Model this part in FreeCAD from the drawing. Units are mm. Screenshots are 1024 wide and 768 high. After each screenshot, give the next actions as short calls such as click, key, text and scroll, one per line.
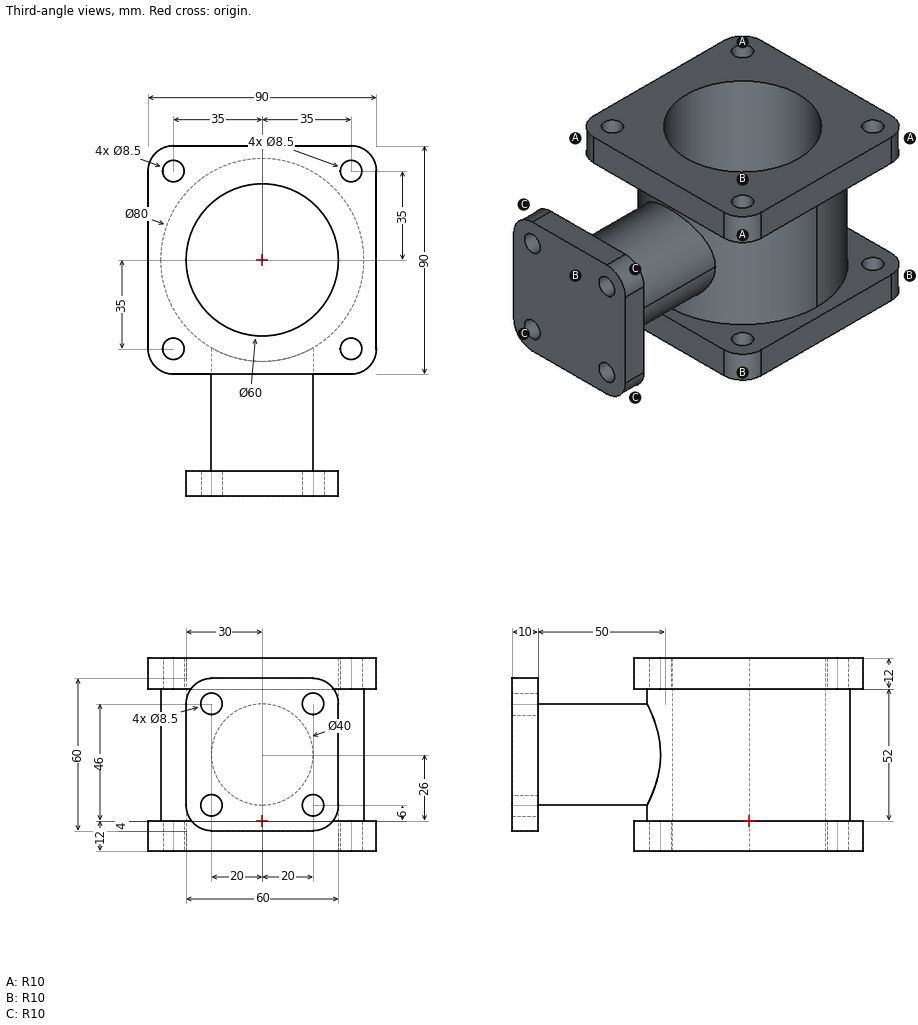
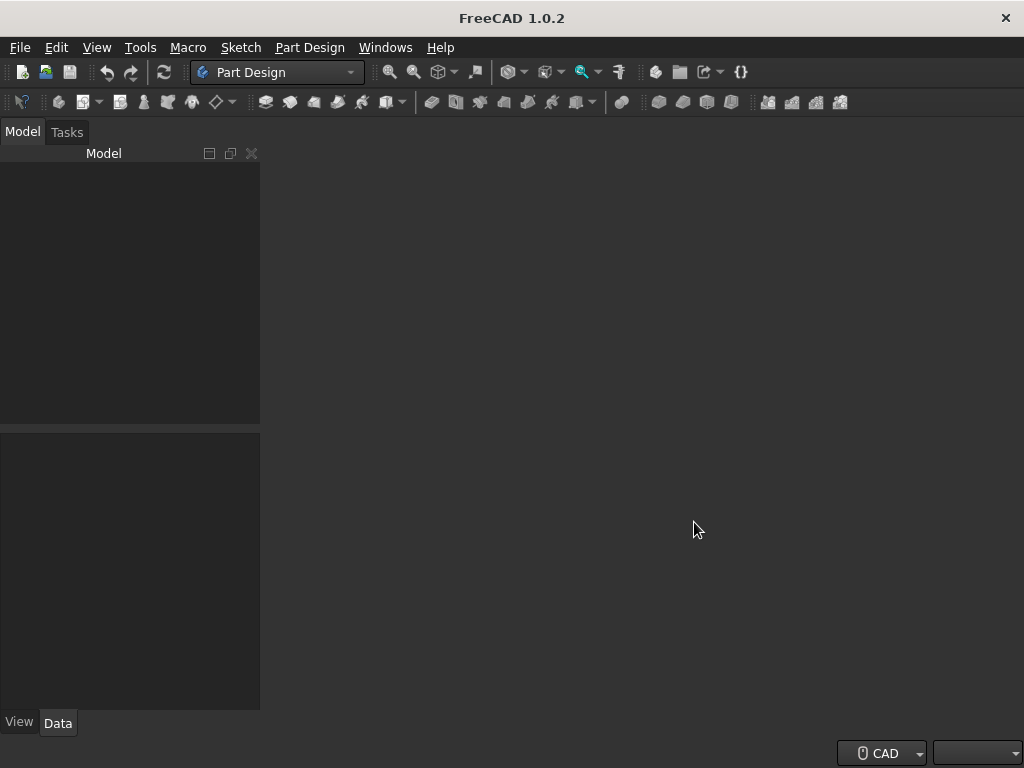
key(ctrl+n)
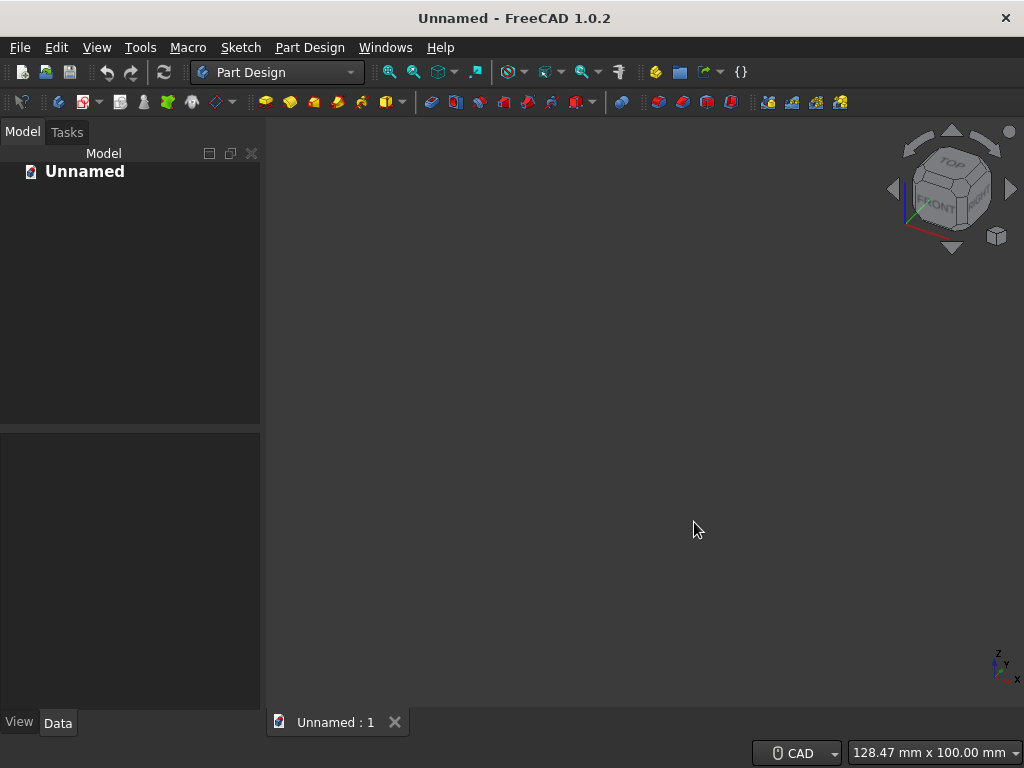
click(84, 102)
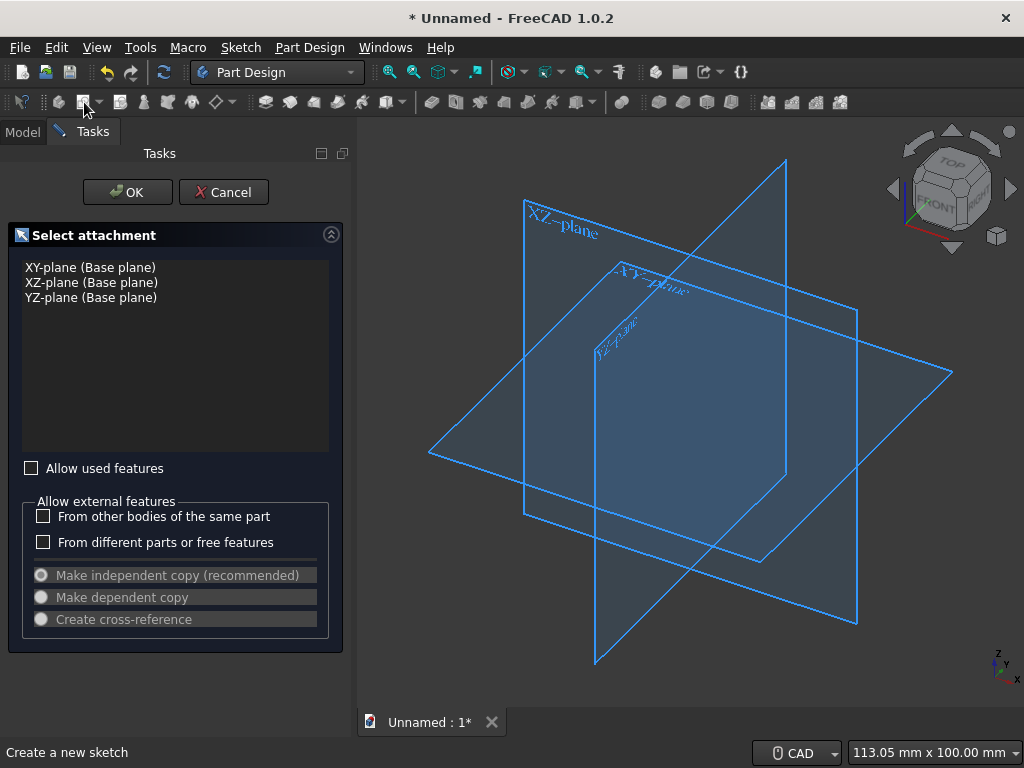
click(82, 268)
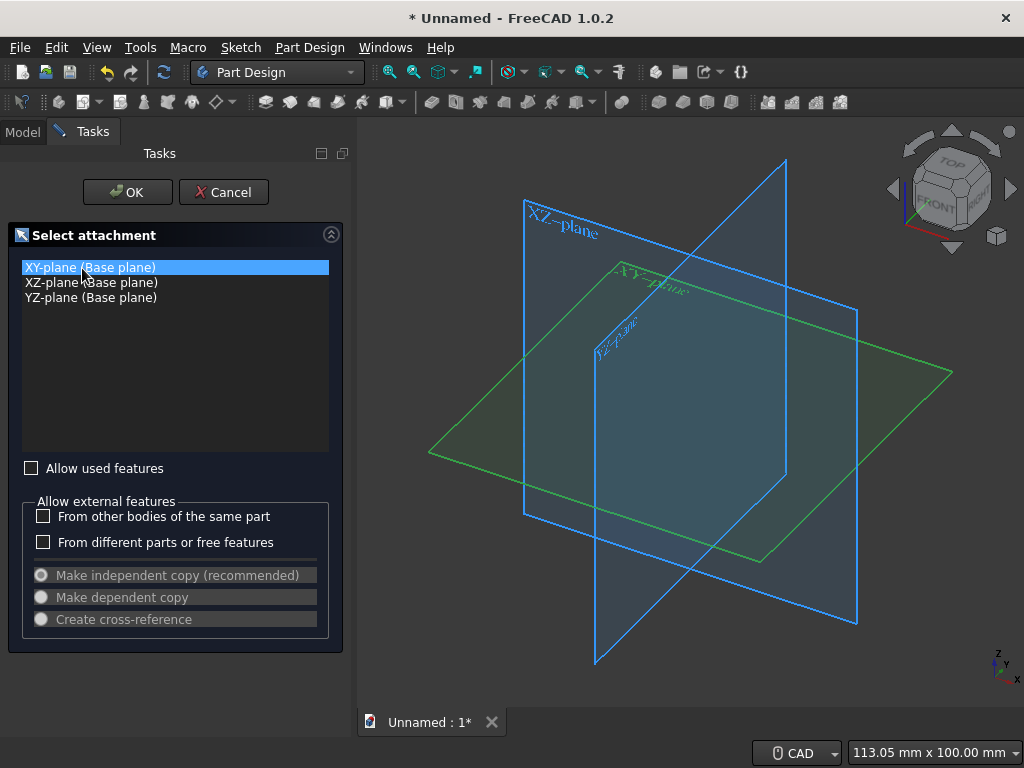
click(128, 192)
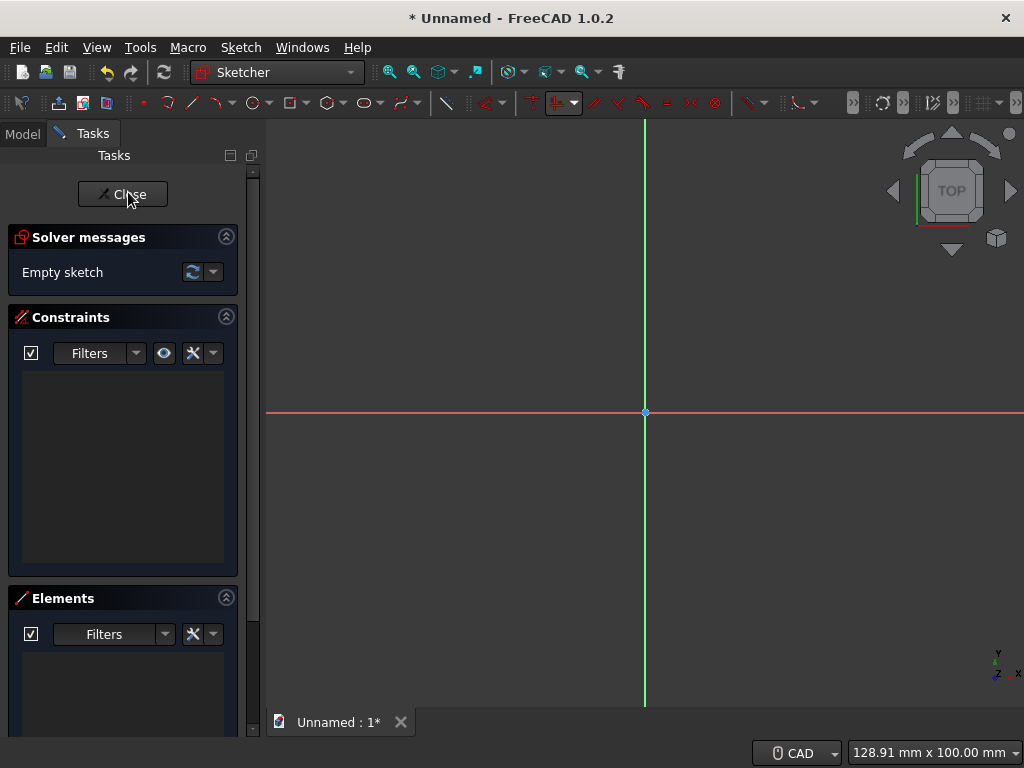
scroll(294, 413, down, 1)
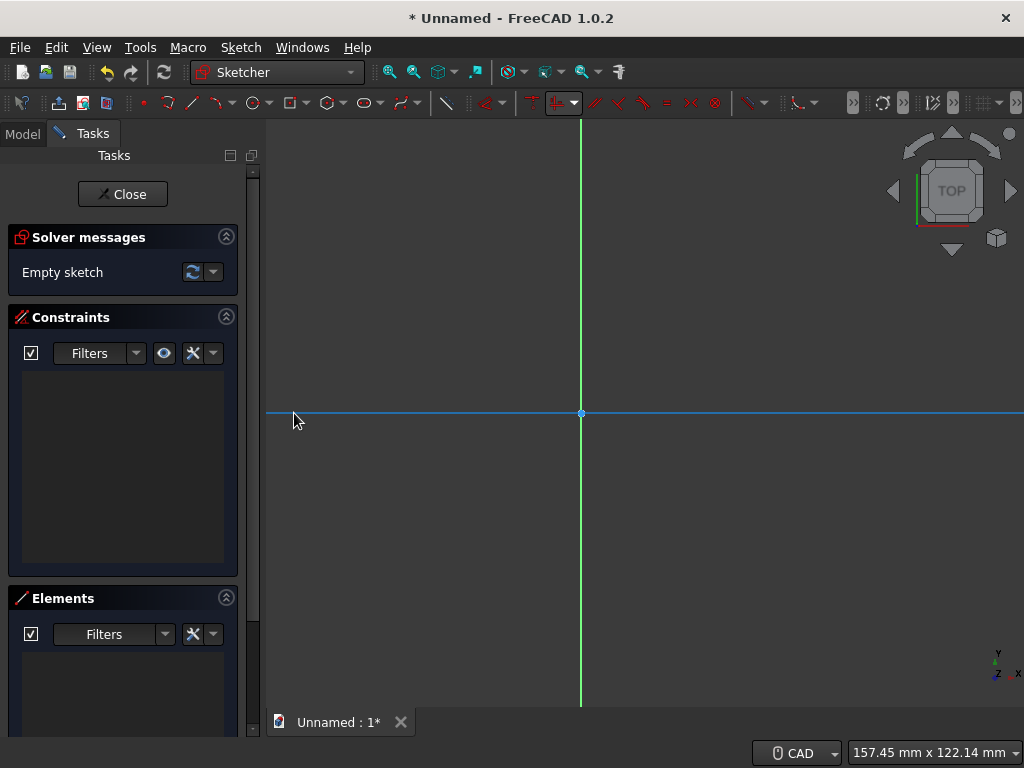
click(254, 104)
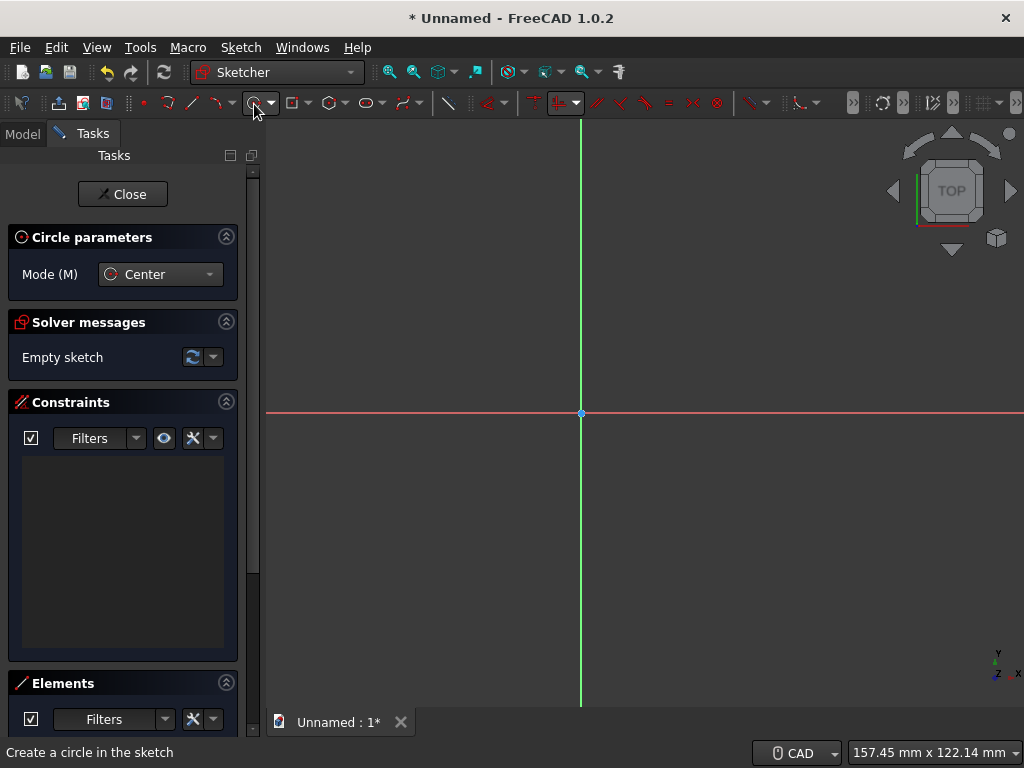
click(581, 413)
click(718, 277)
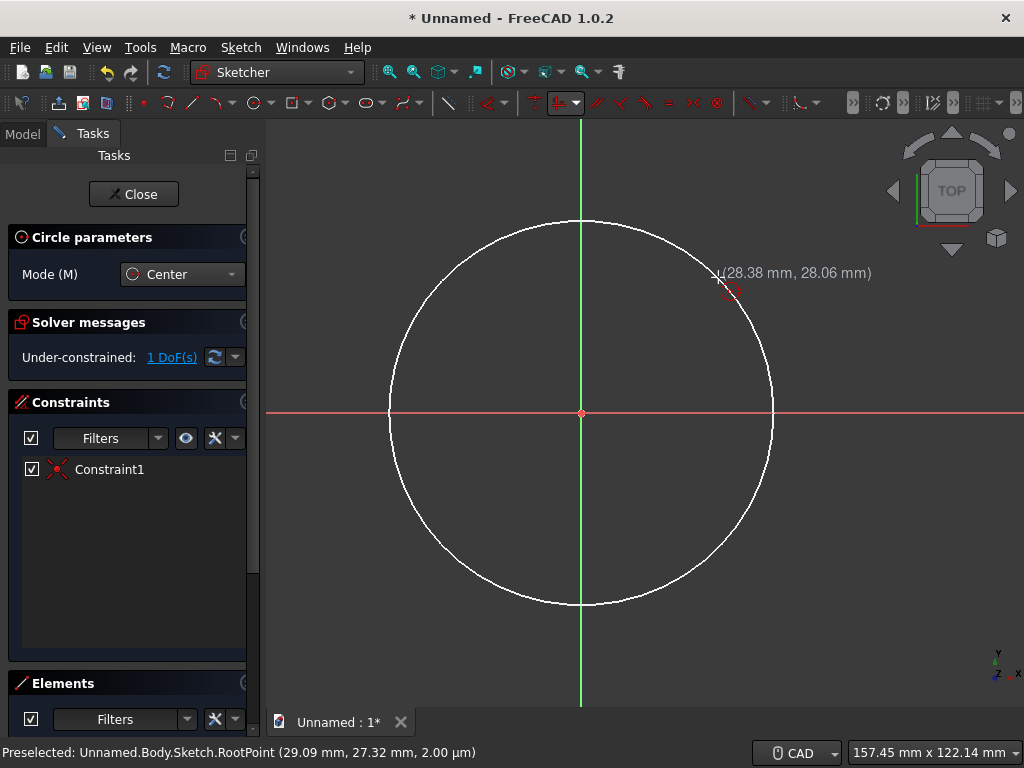
click(581, 413)
click(684, 311)
key(Escape)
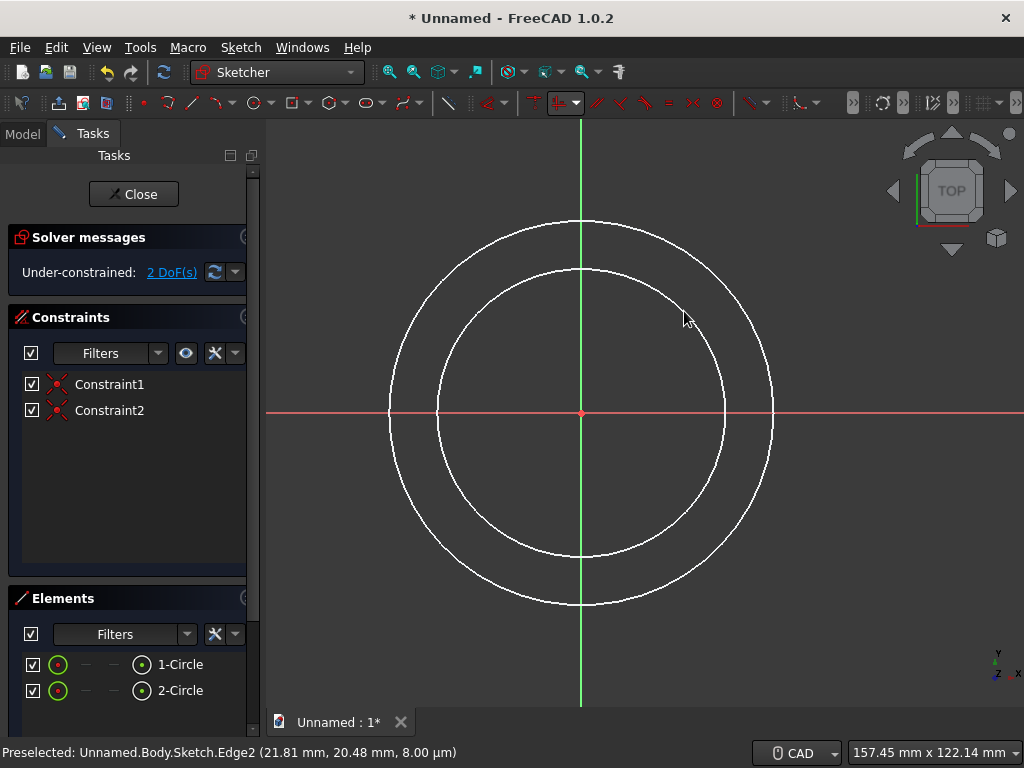
click(488, 104)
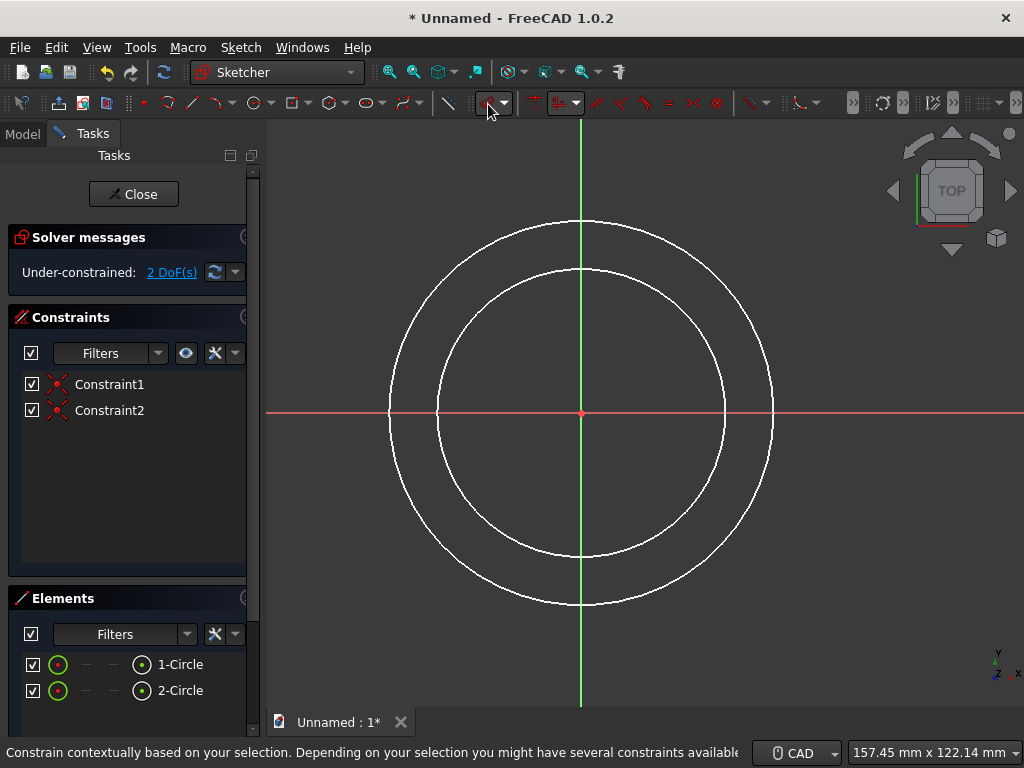
click(717, 277)
click(740, 254)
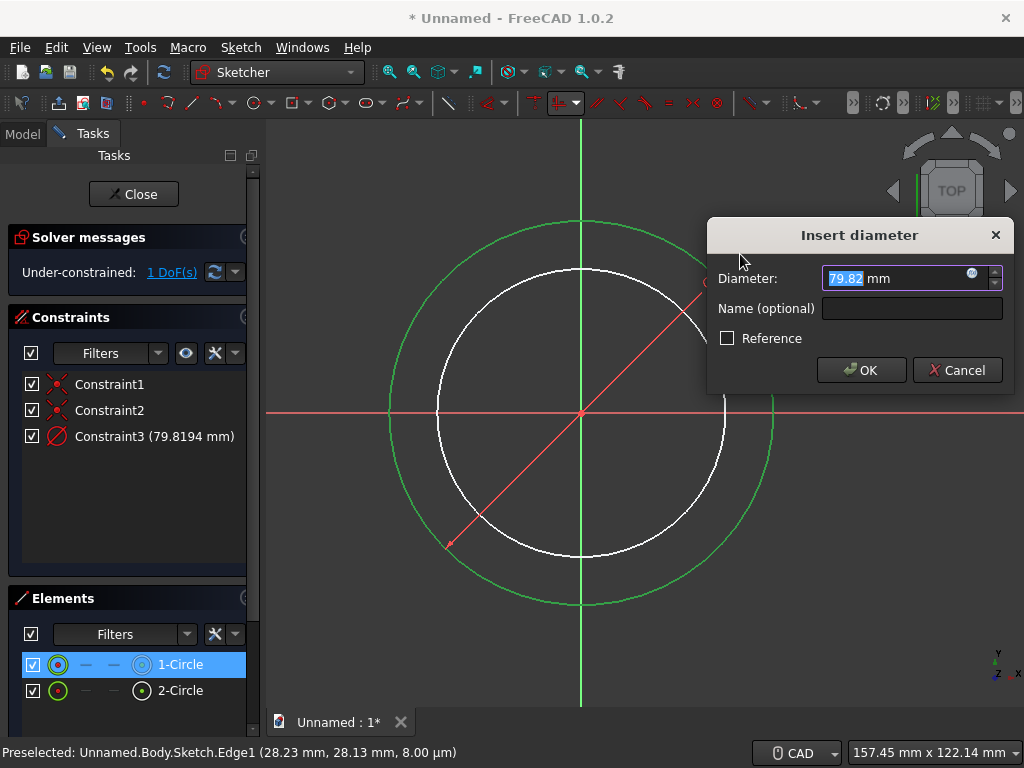
text(80)
key(Return)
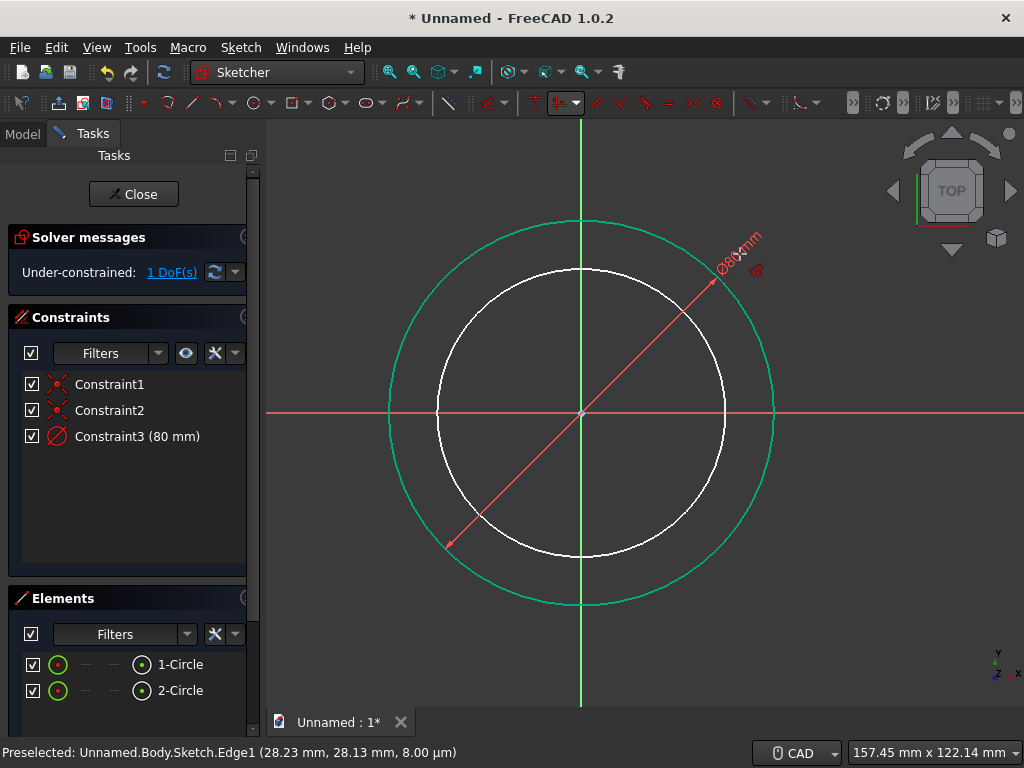
click(683, 311)
click(706, 288)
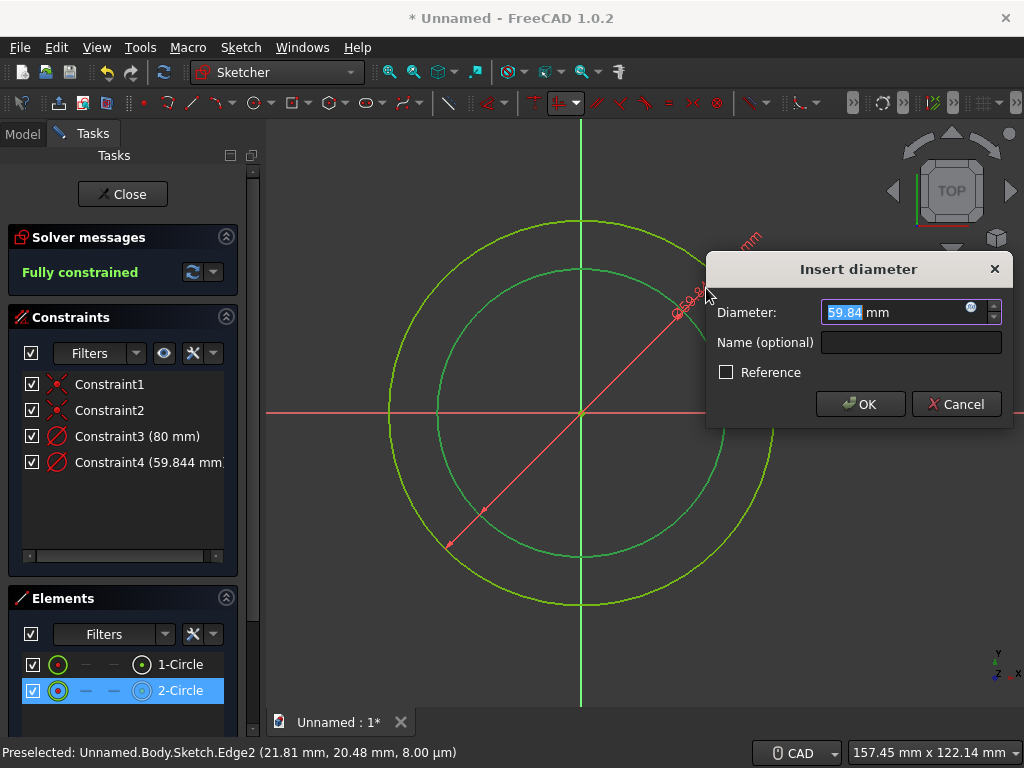
text(60)
key(Return)
key(Escape)